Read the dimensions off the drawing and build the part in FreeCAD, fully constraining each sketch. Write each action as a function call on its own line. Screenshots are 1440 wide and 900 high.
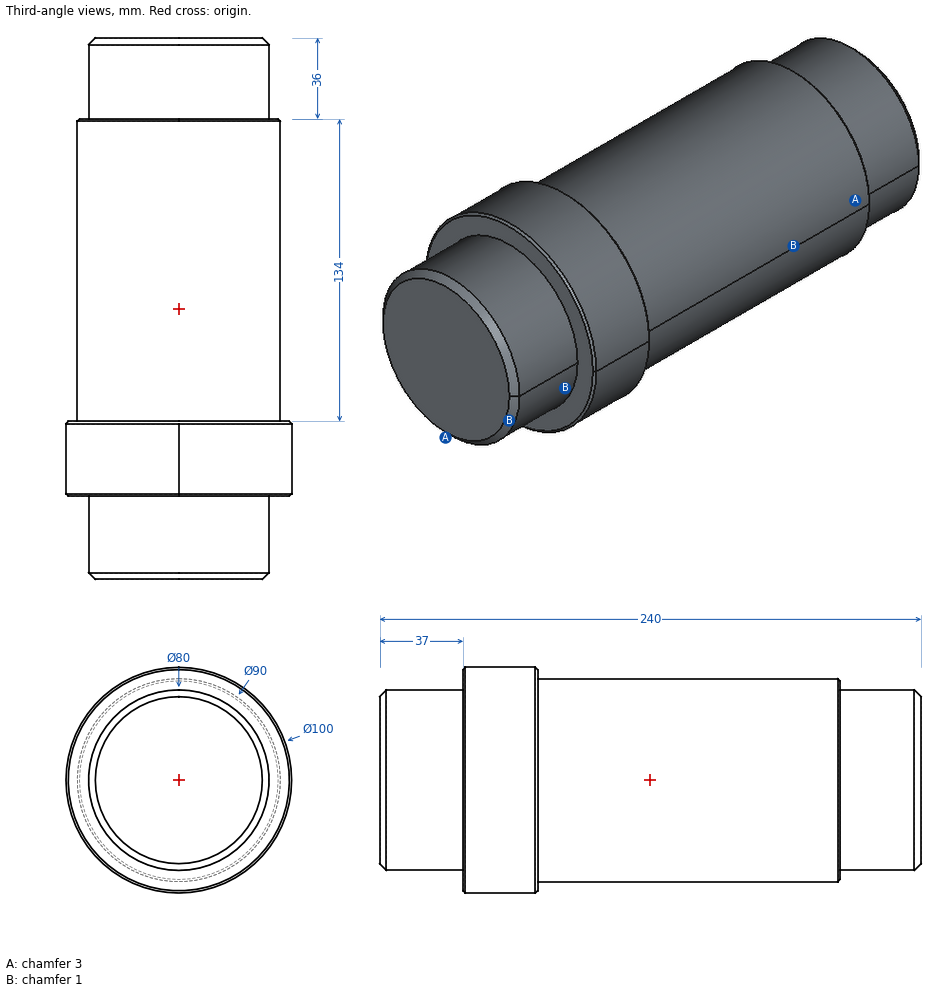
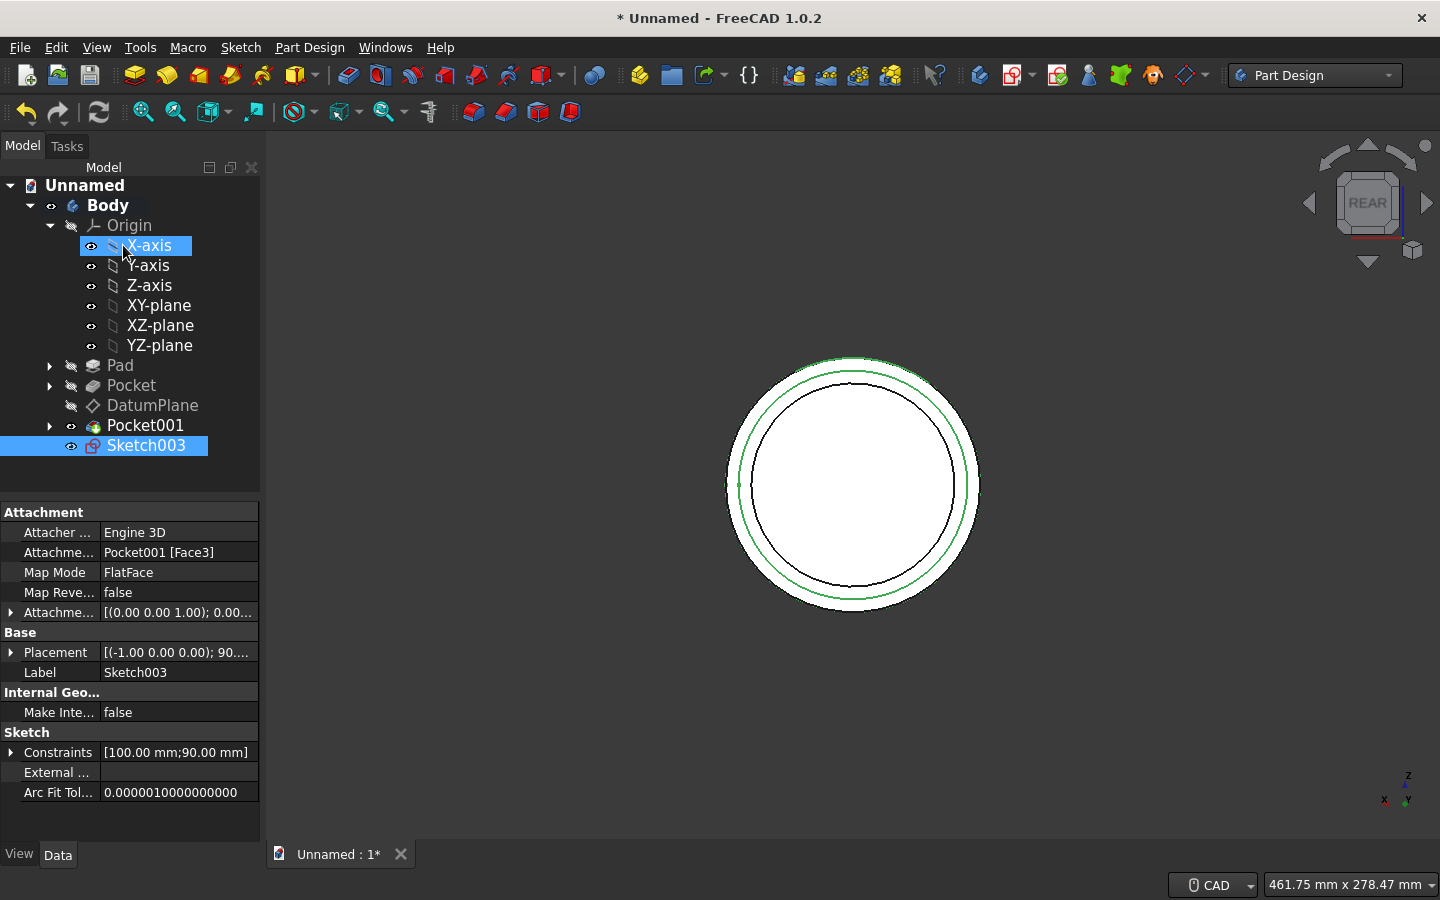
click(350, 76)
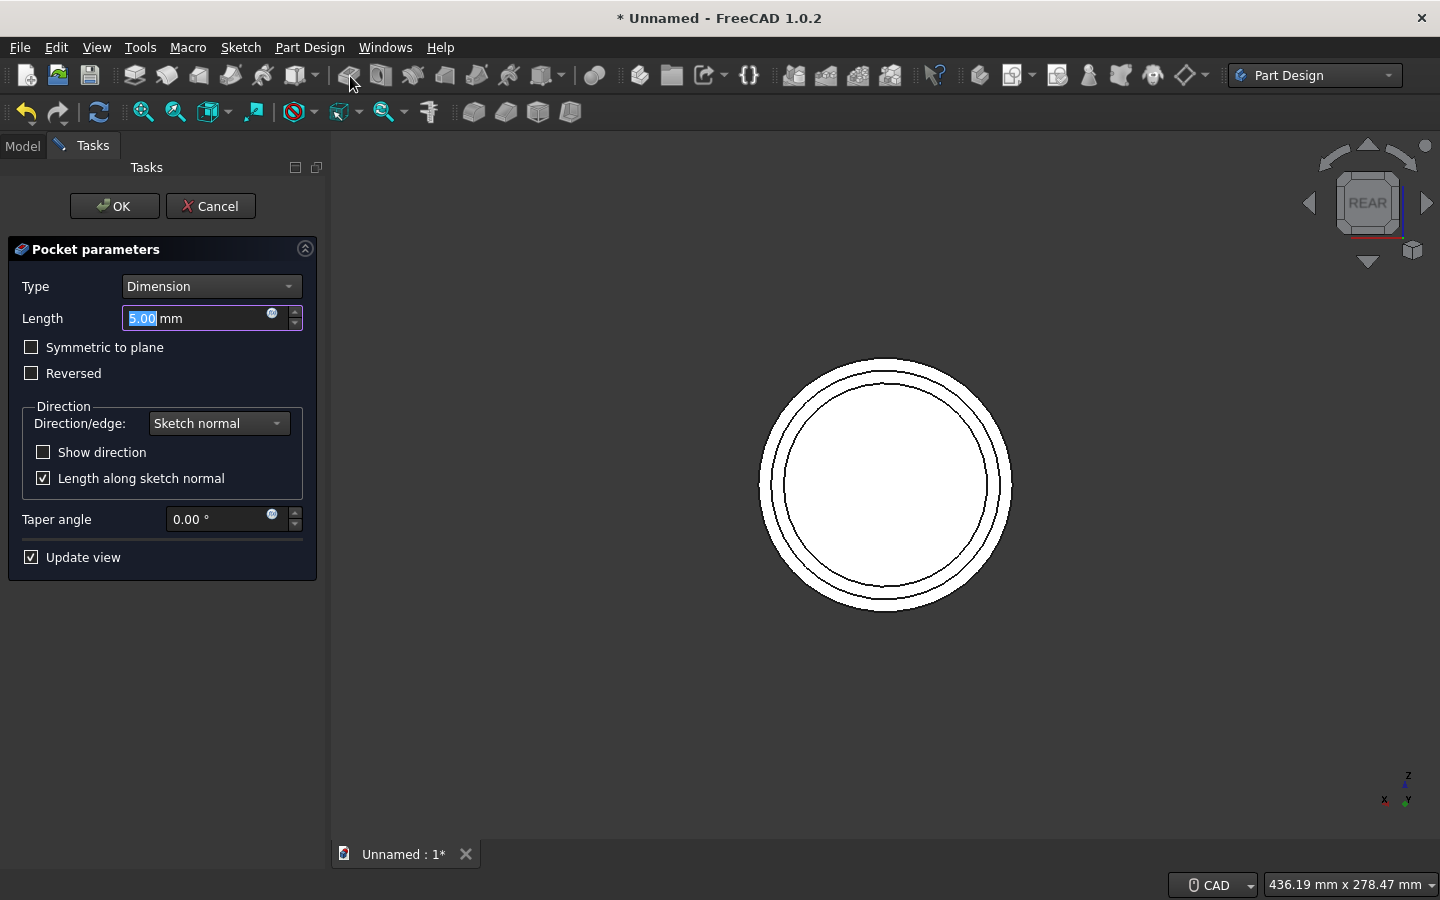
text(134)
key(Tab)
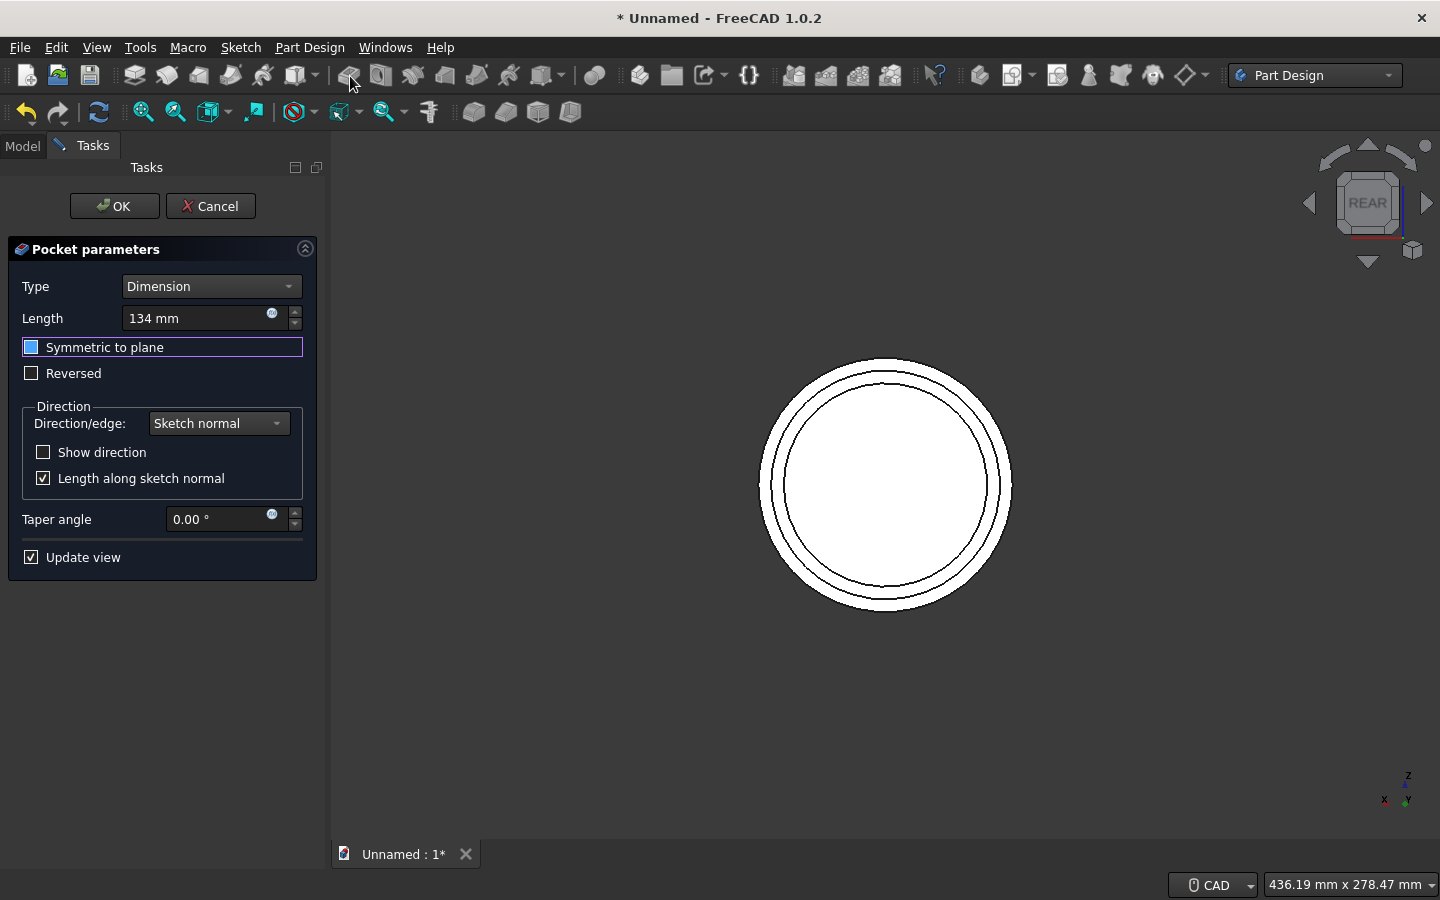
click(115, 206)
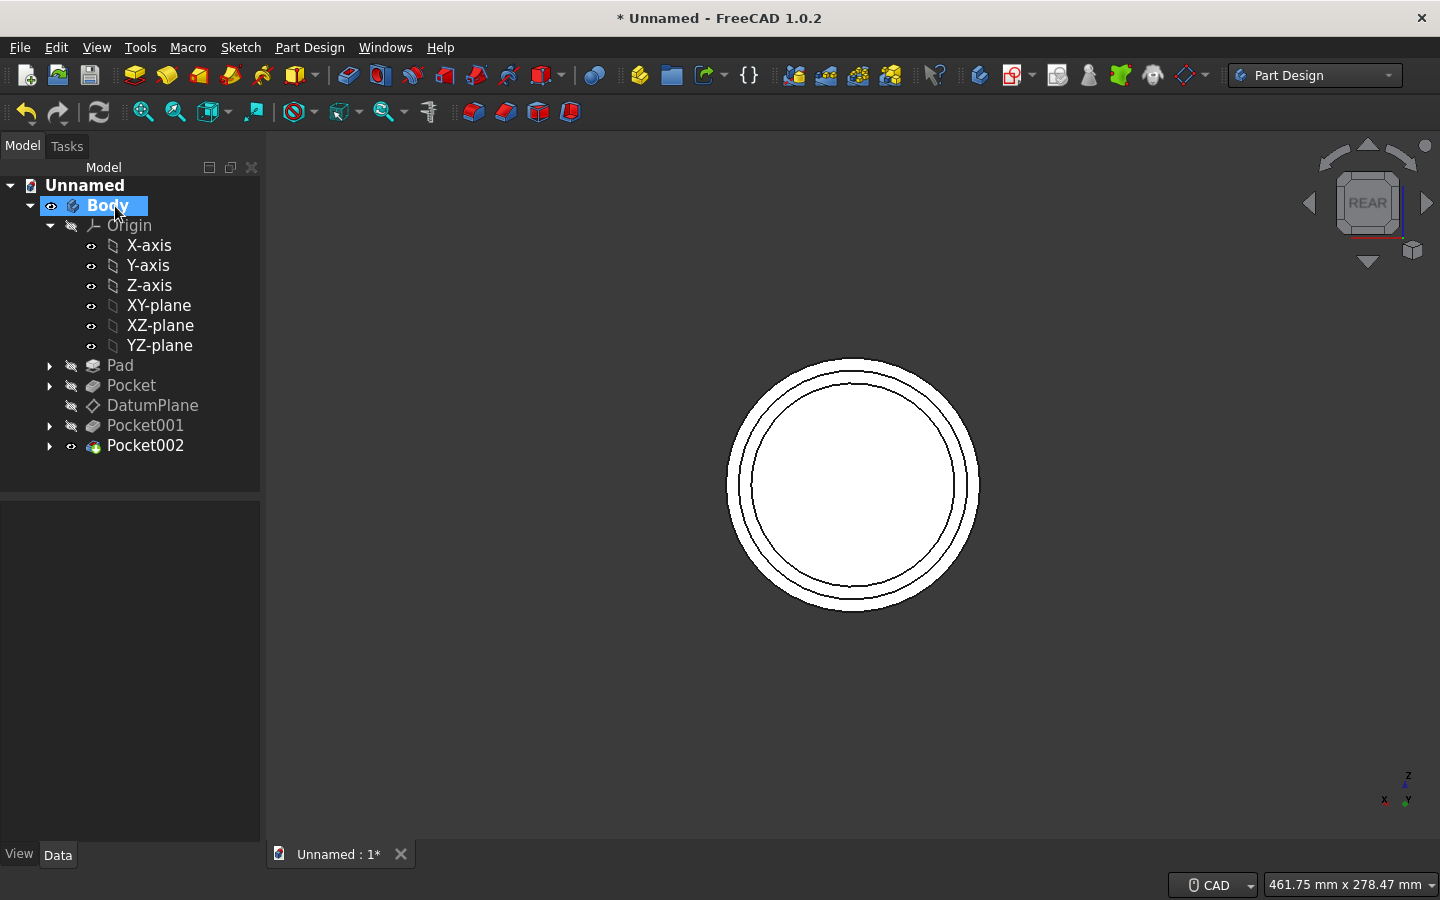
click(144, 112)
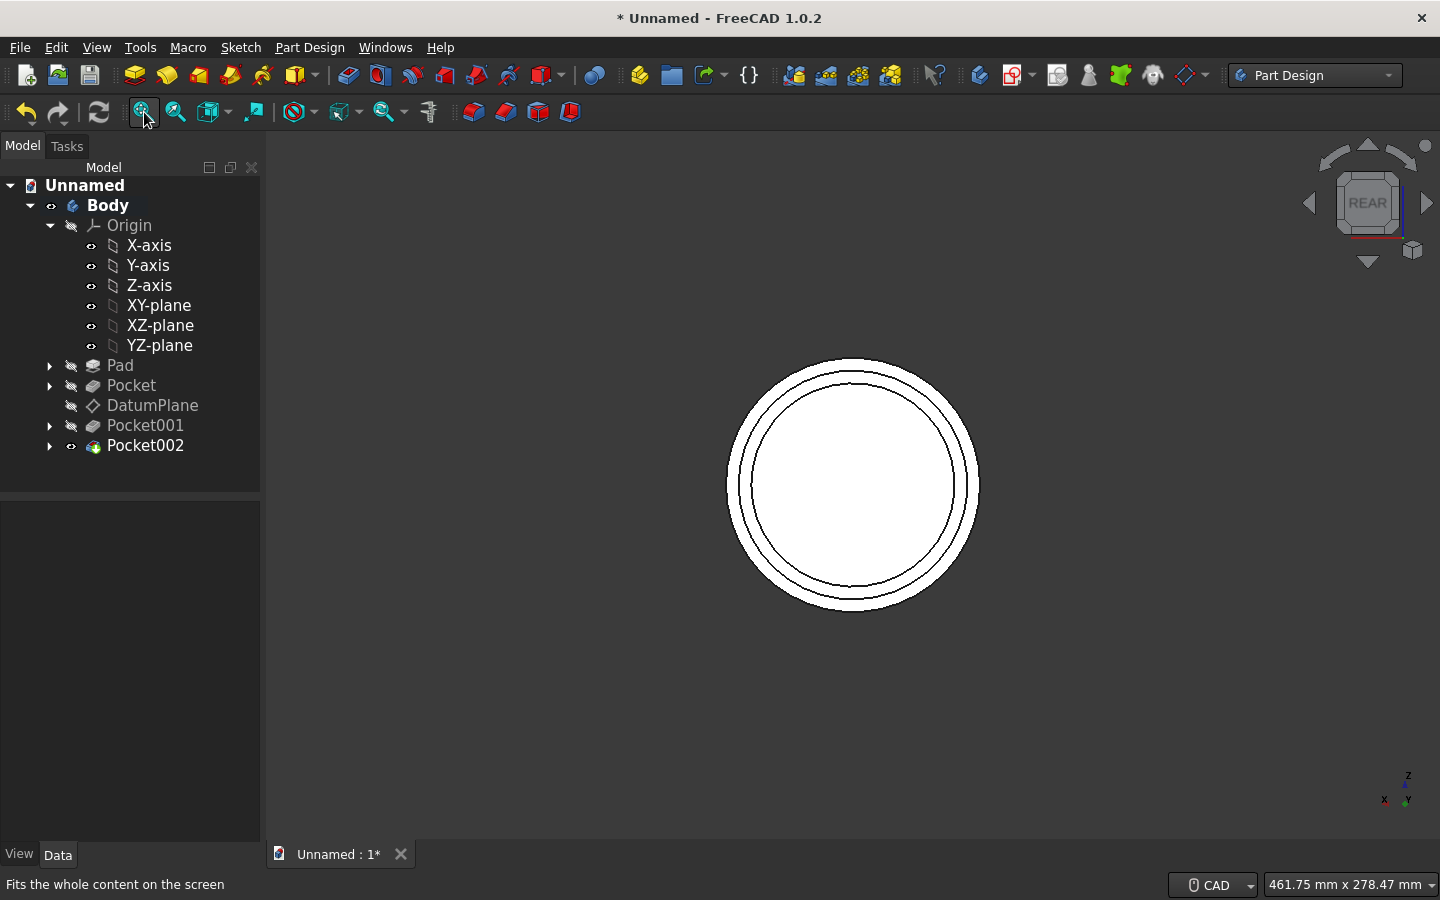
click(955, 484)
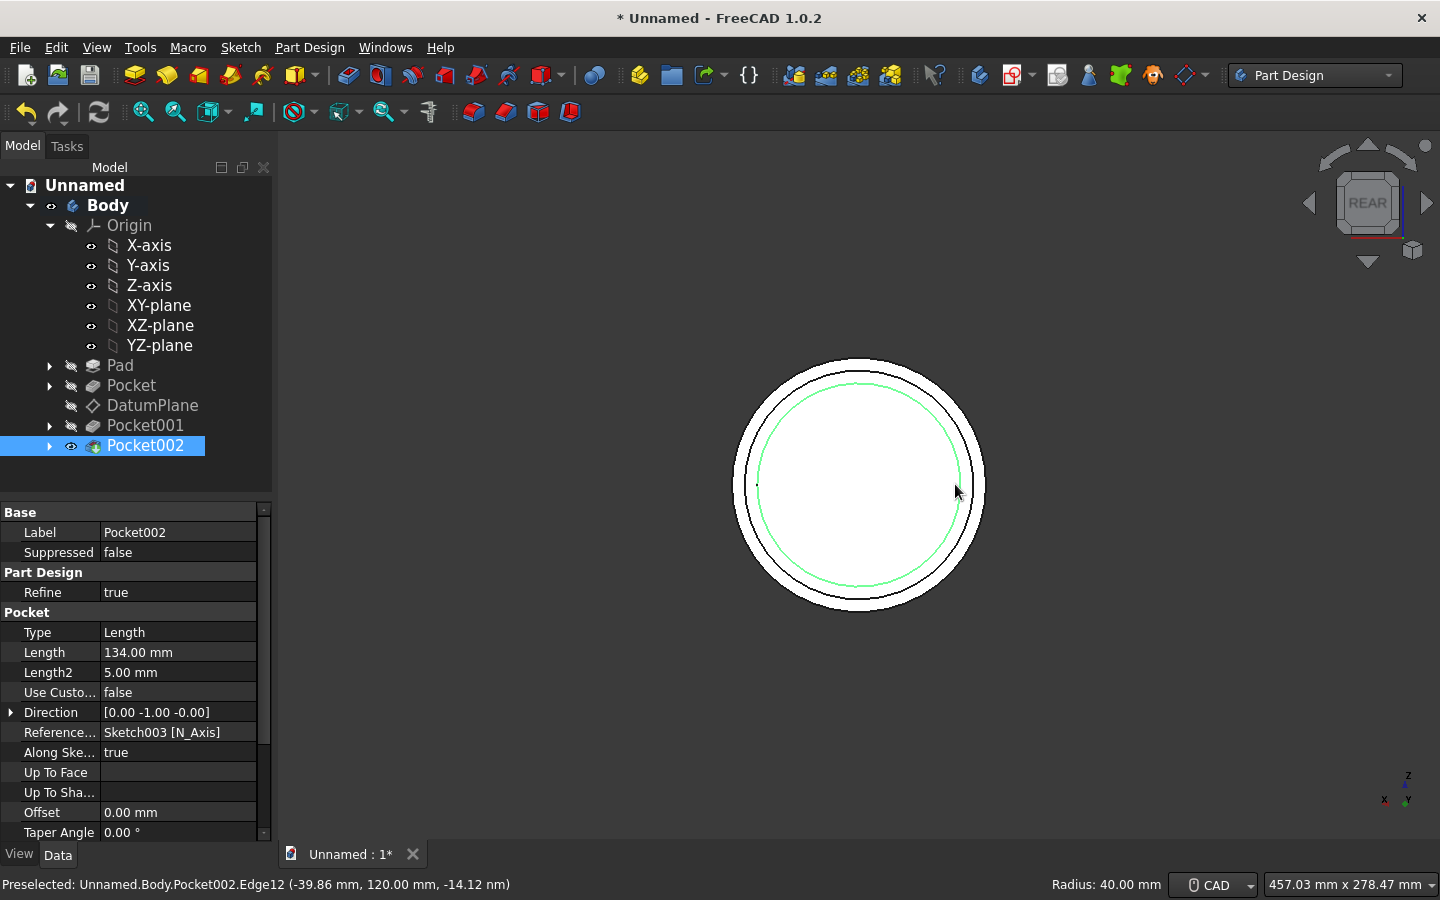
key(0)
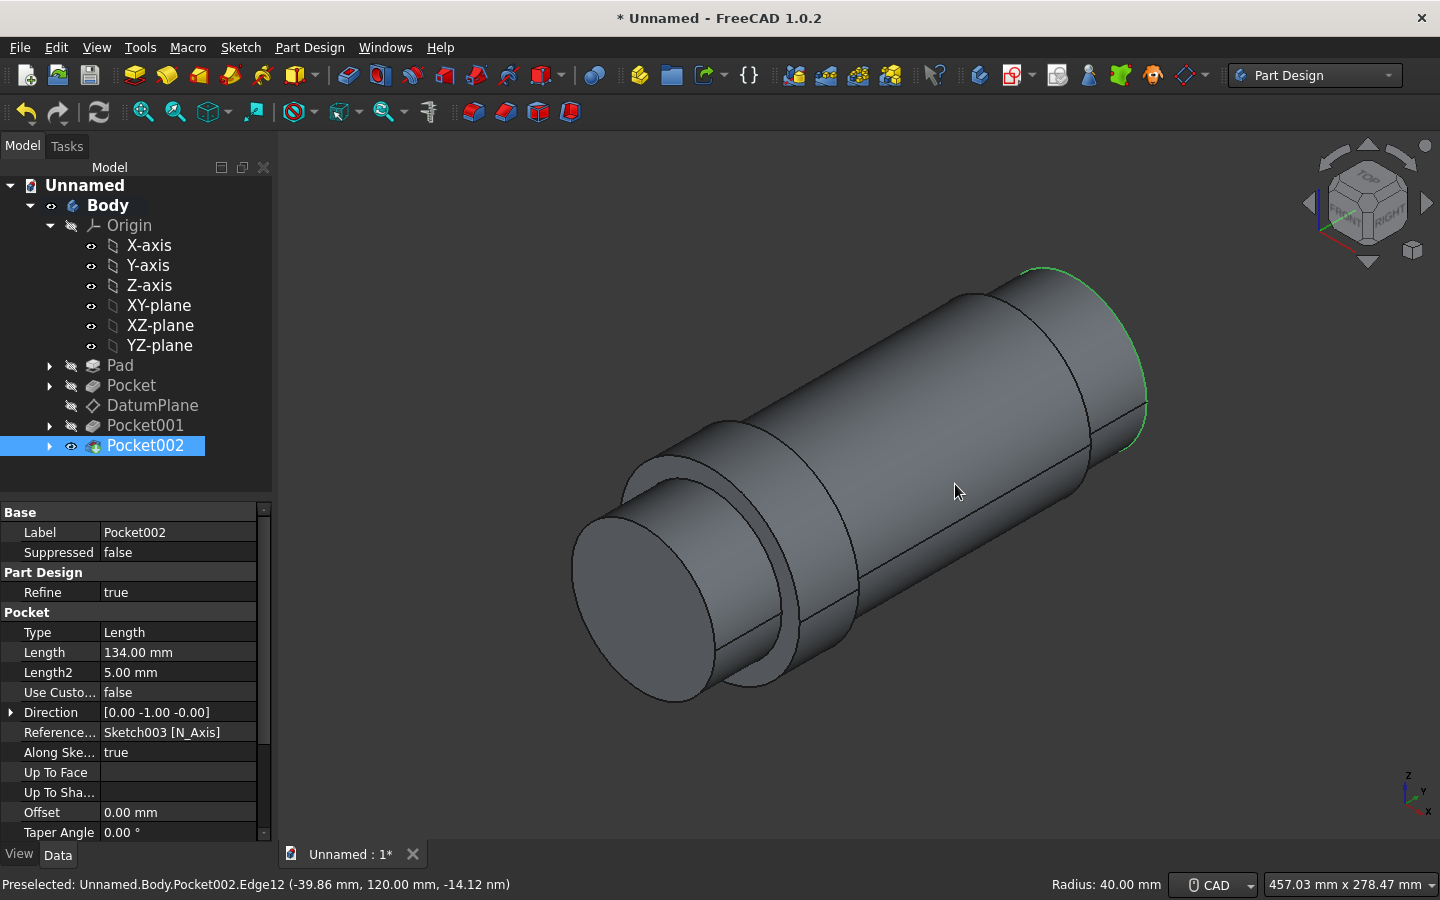
click(621, 517, ctrl)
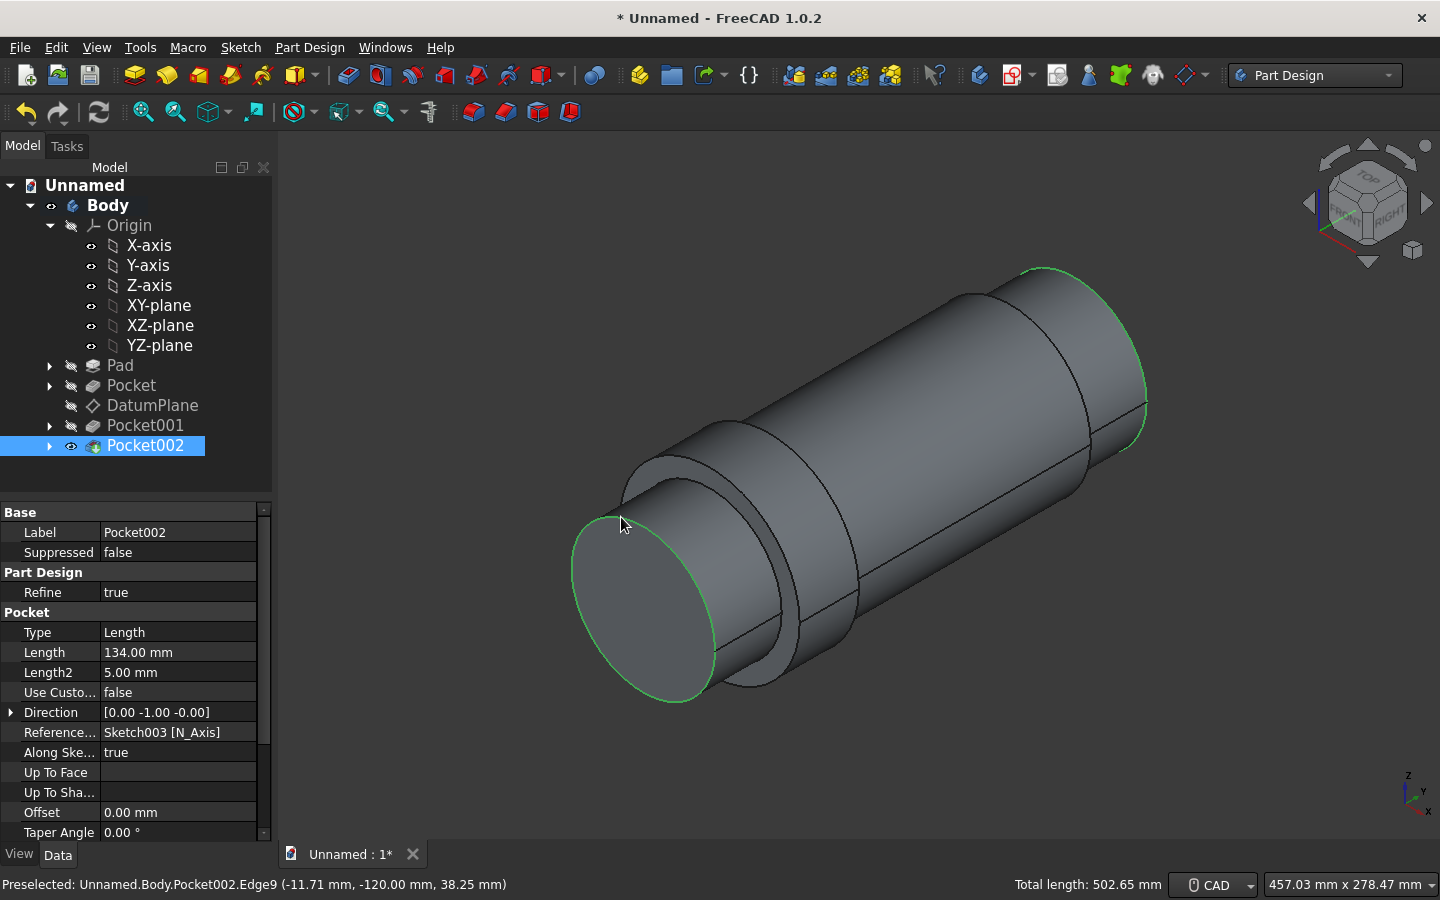
click(506, 112)